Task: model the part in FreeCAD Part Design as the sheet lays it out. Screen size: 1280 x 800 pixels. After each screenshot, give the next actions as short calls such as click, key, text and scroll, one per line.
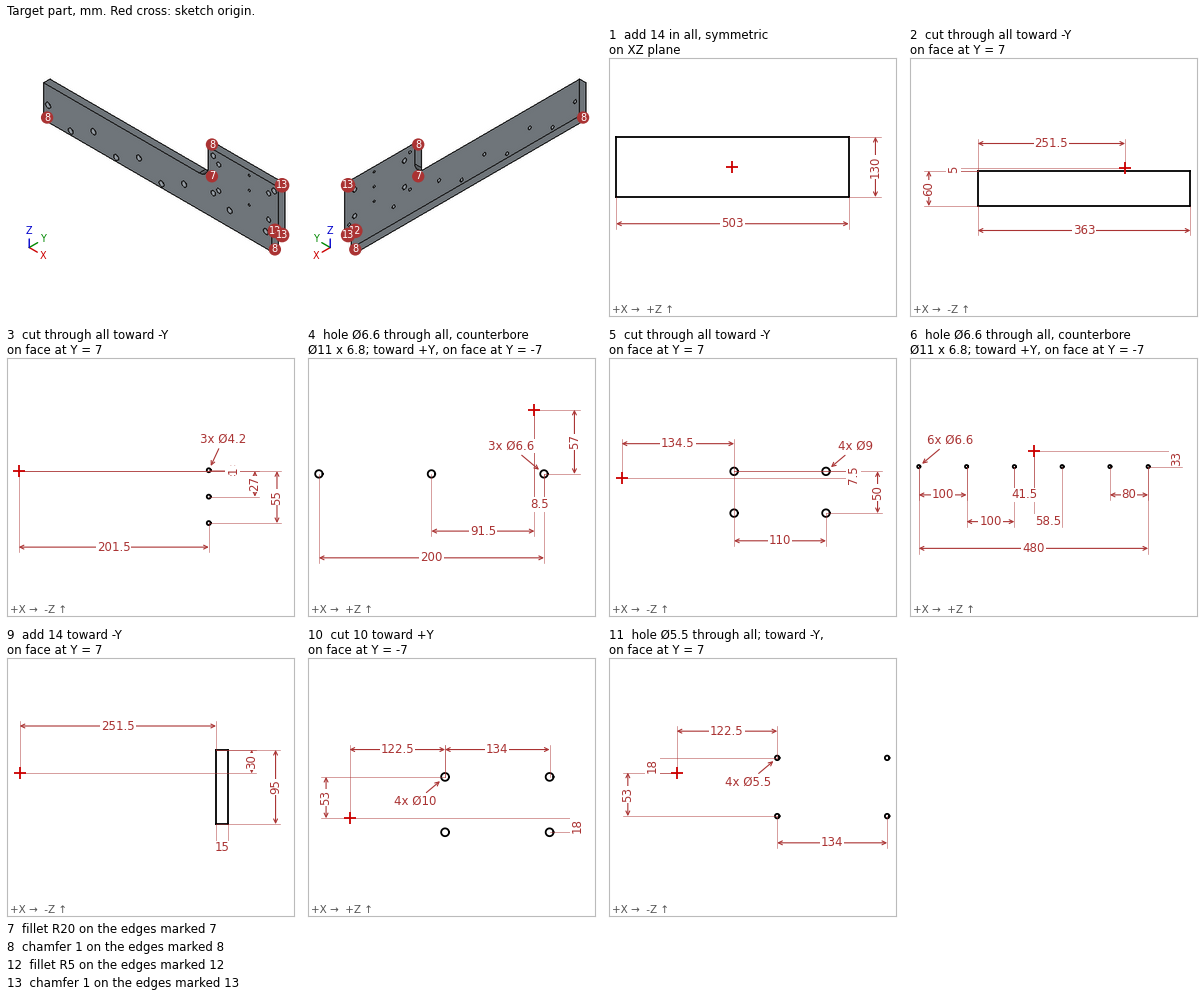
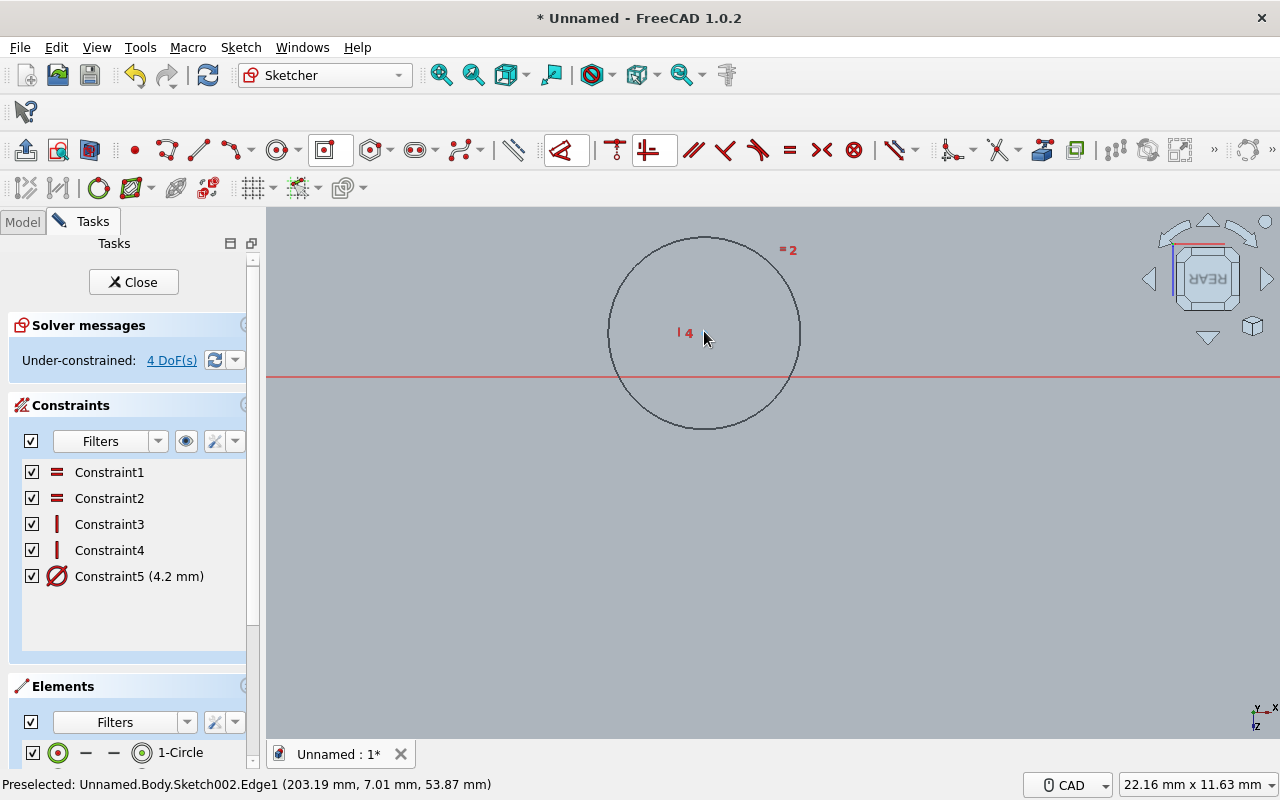
click(704, 333)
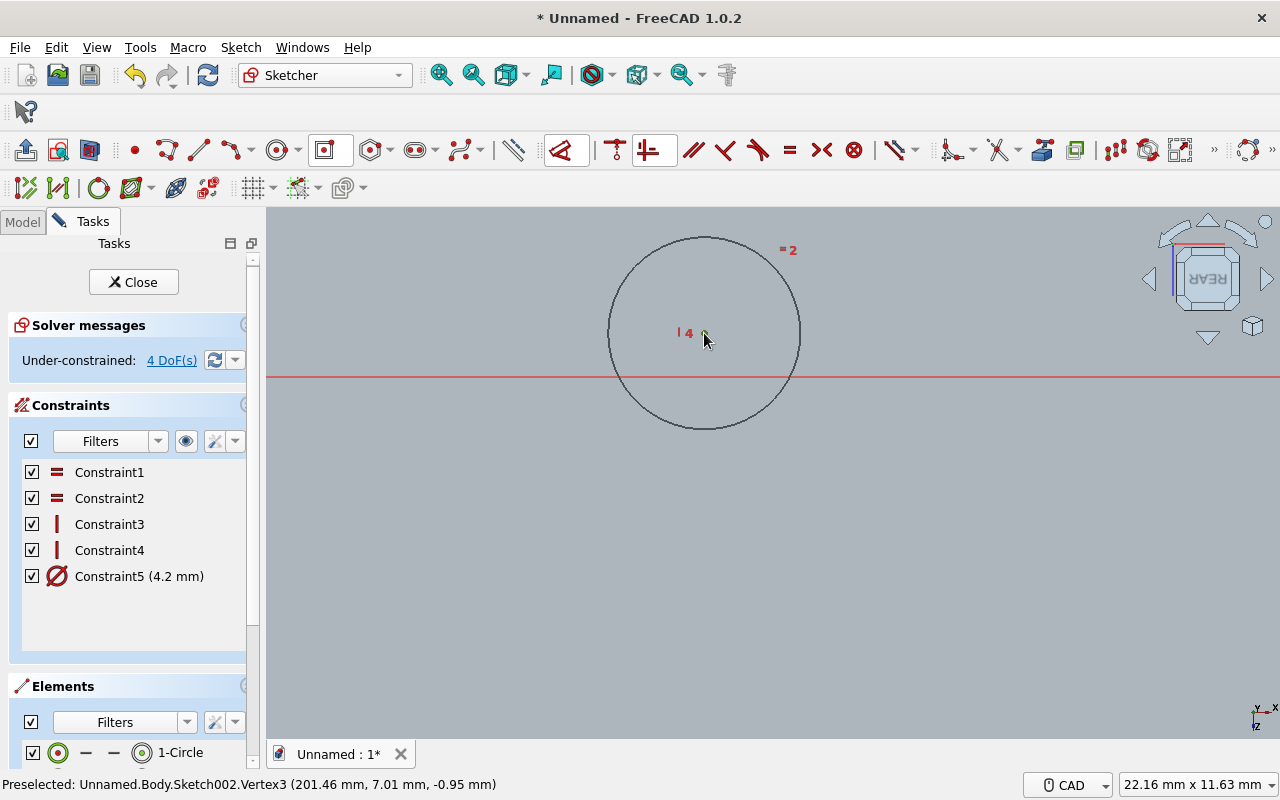
click(584, 150)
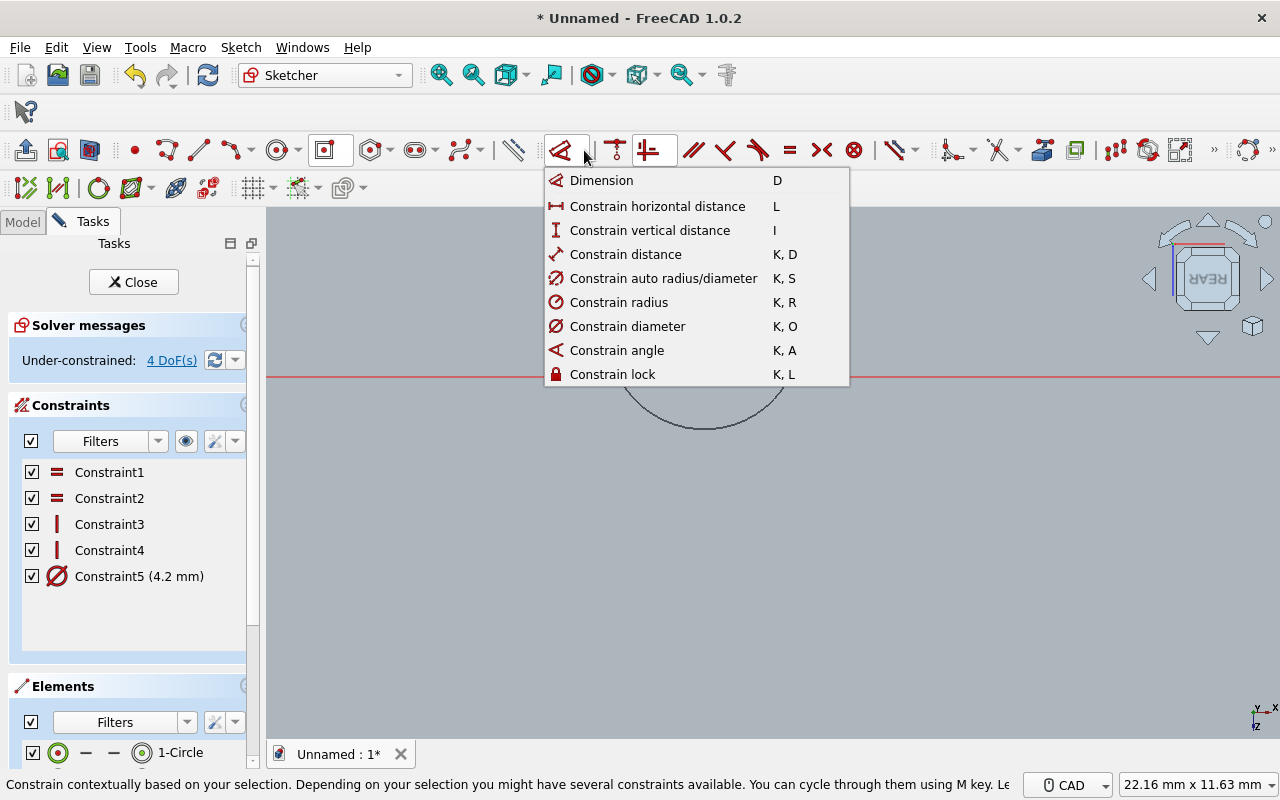
click(697, 230)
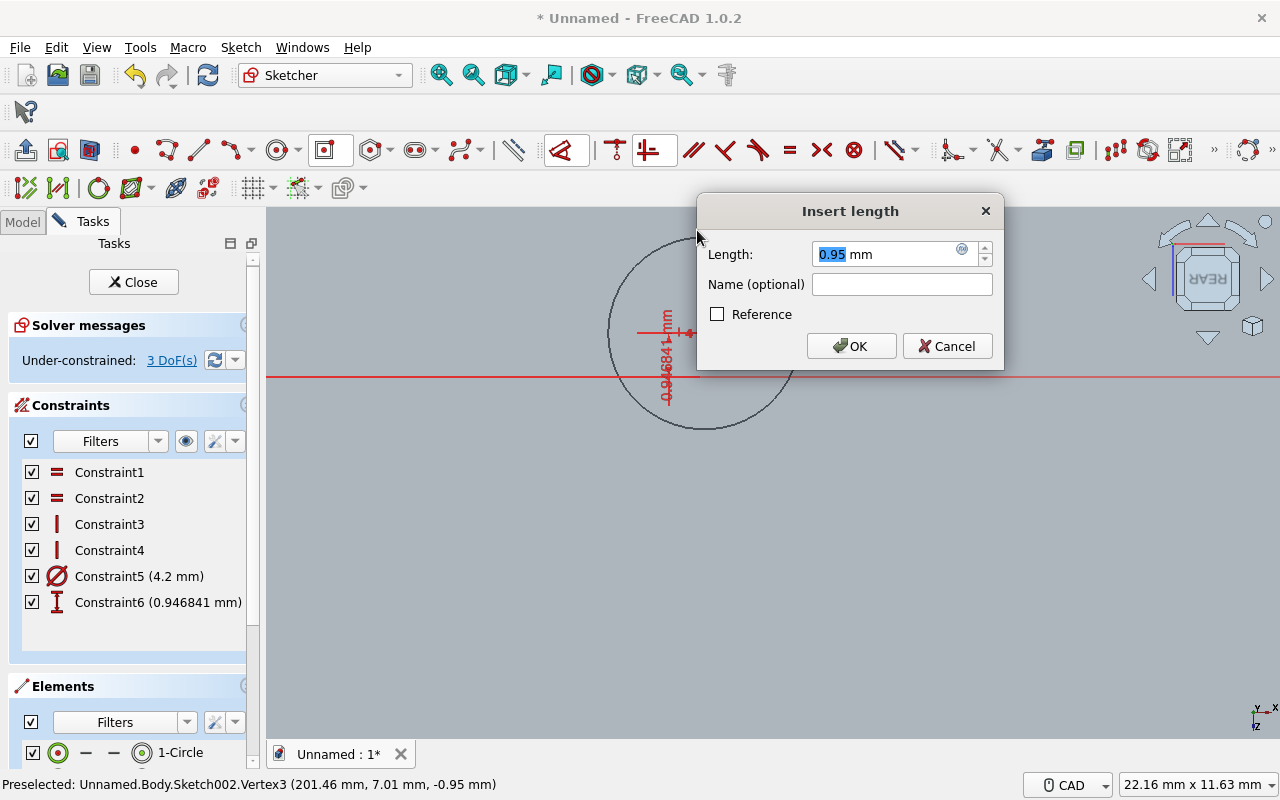
text(1)
key(Return)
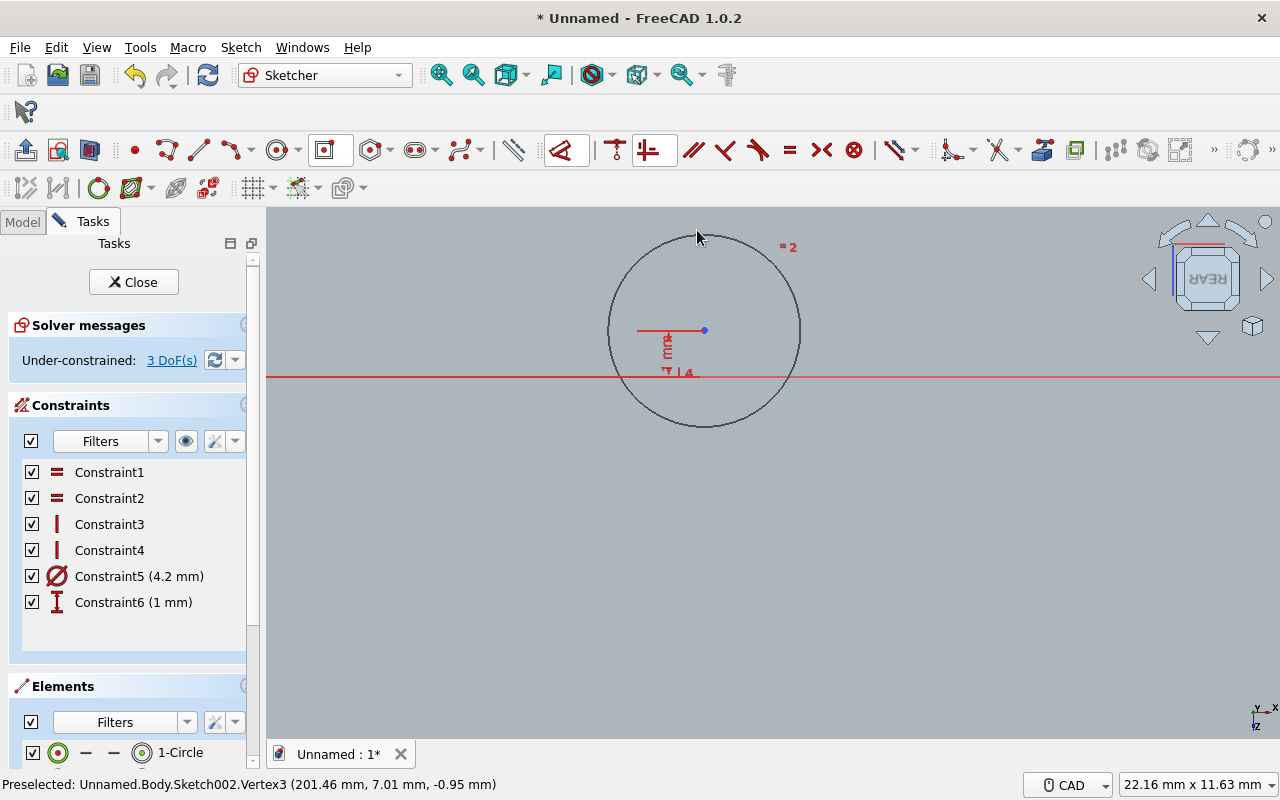
scroll(704, 331, down, 11)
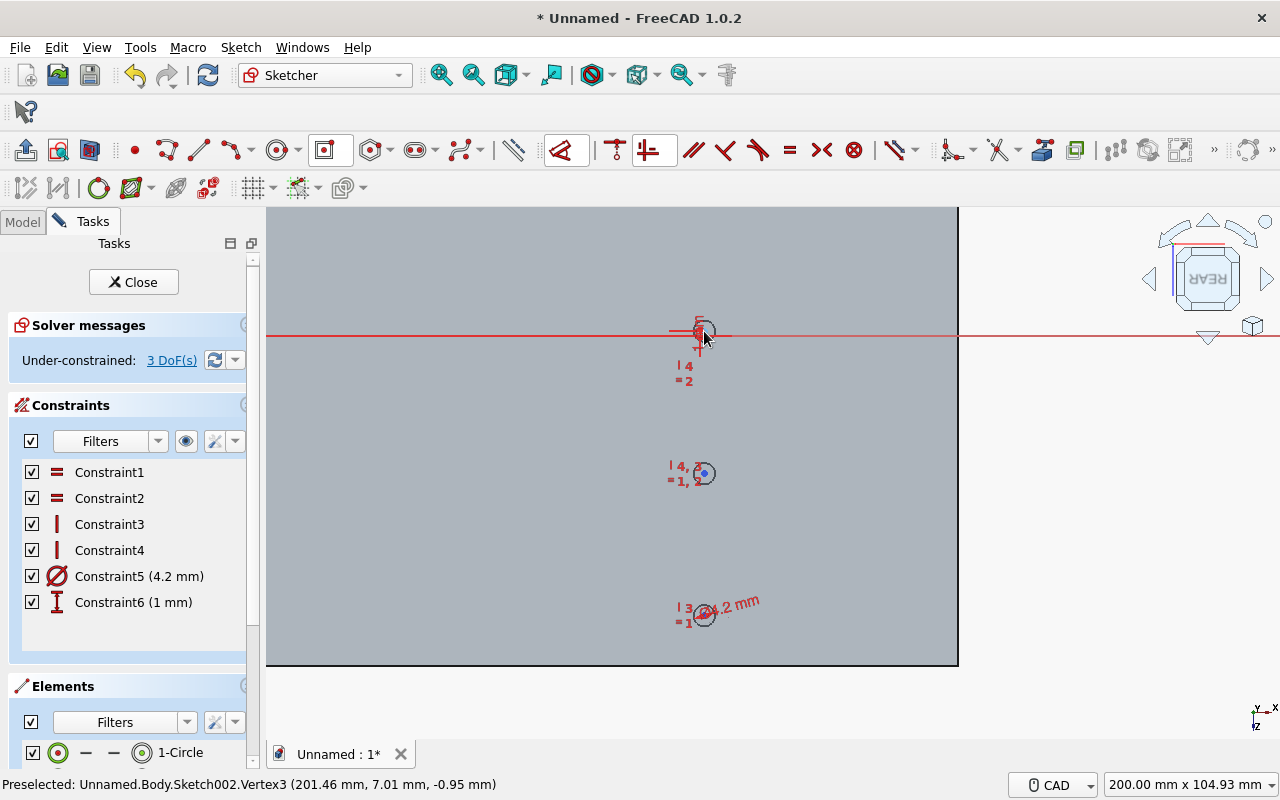
click(704, 616)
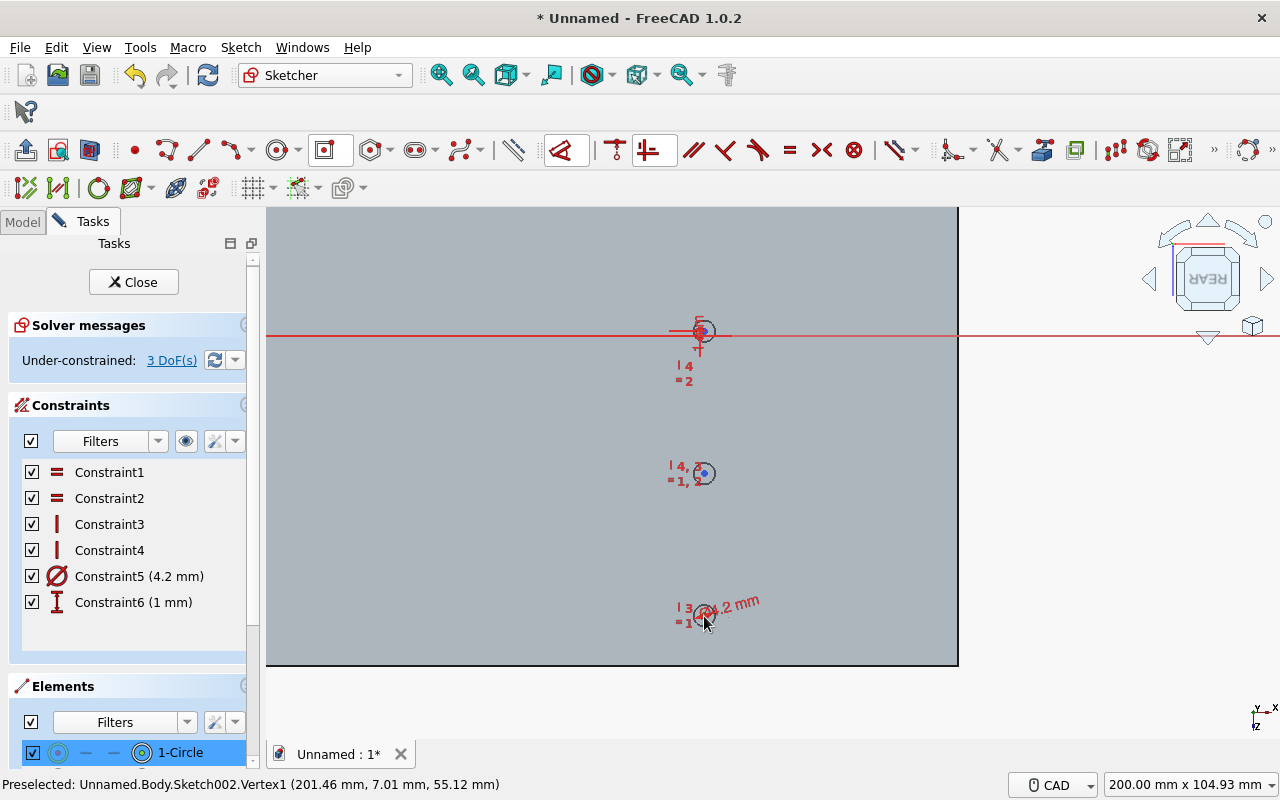
click(584, 150)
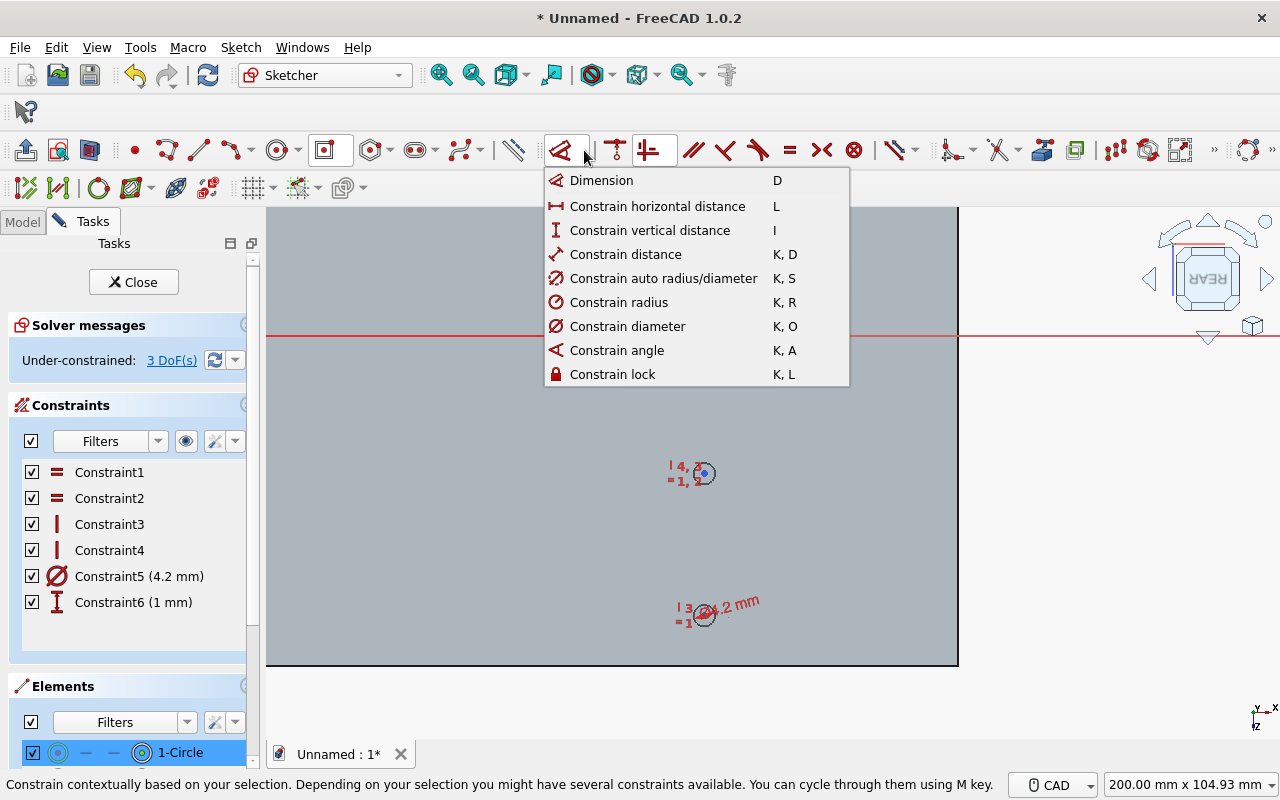
click(697, 230)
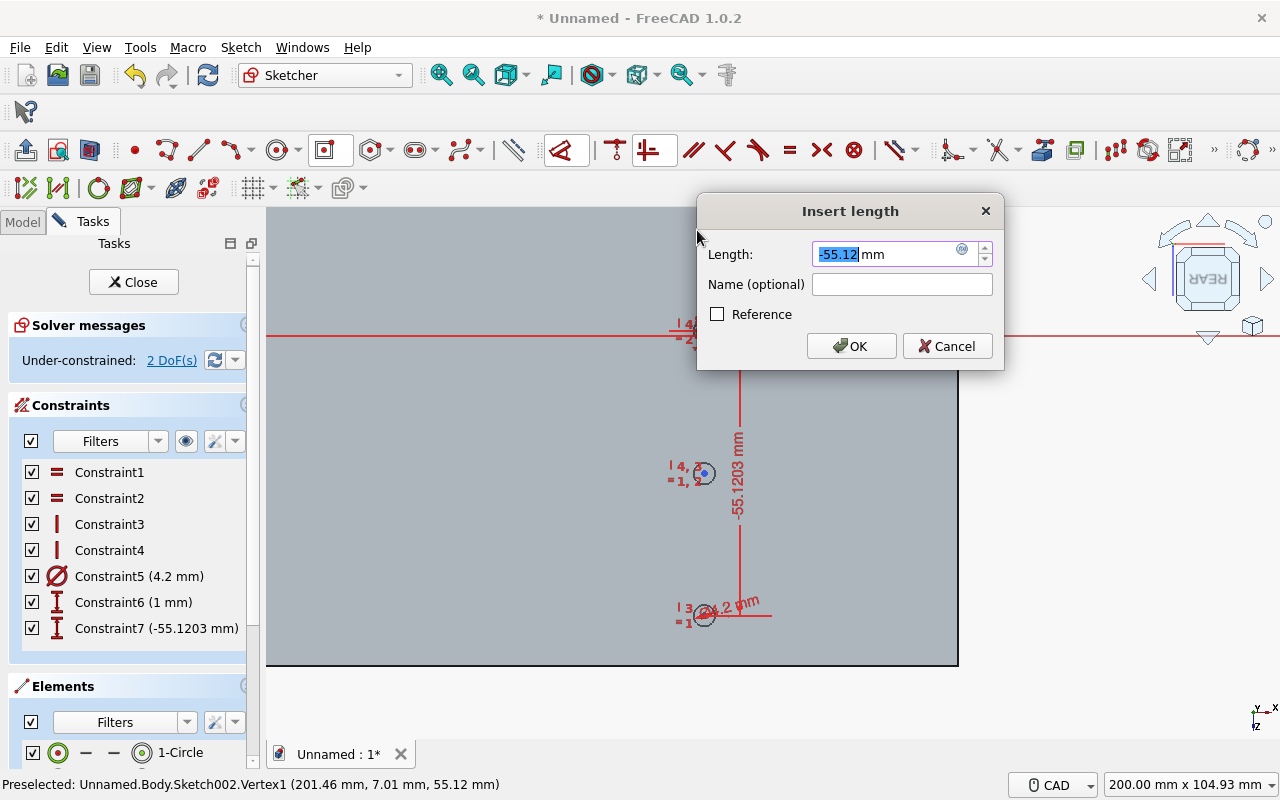
text(-55)
key(Return)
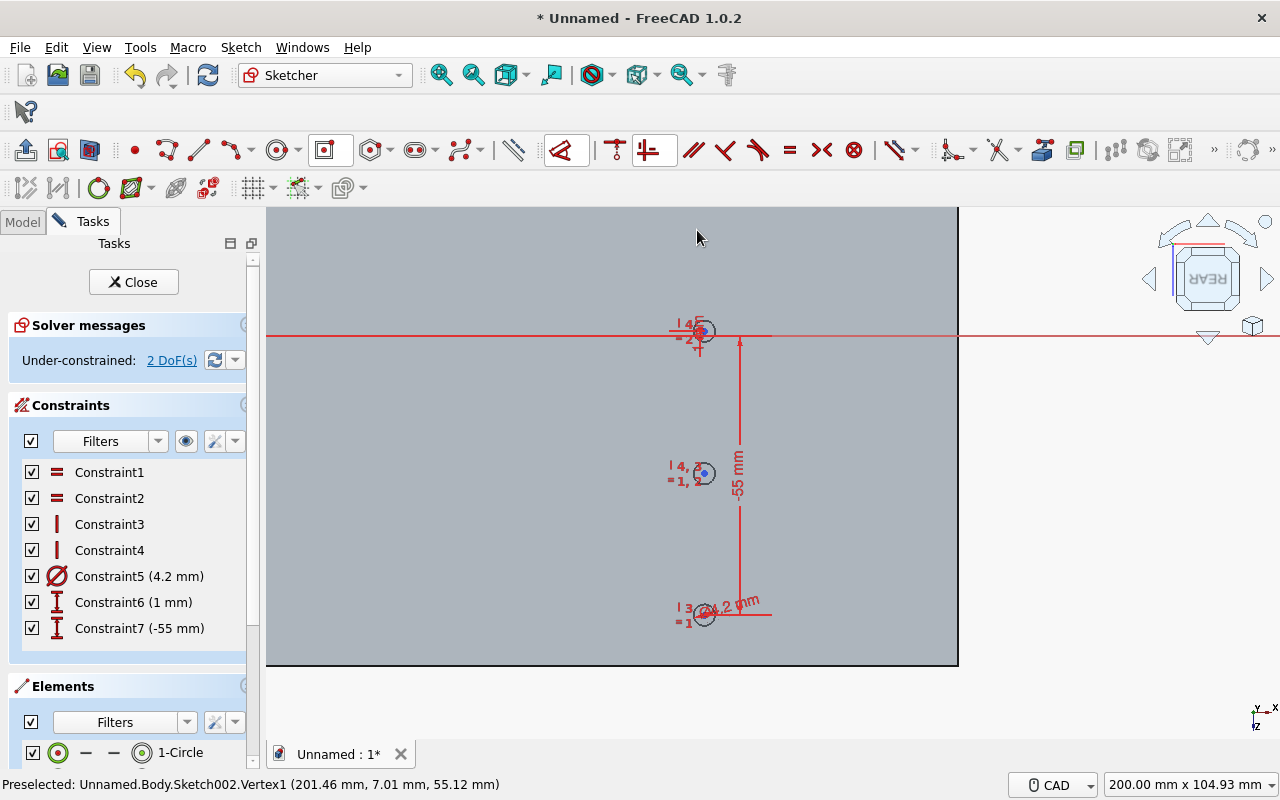
click(704, 474)